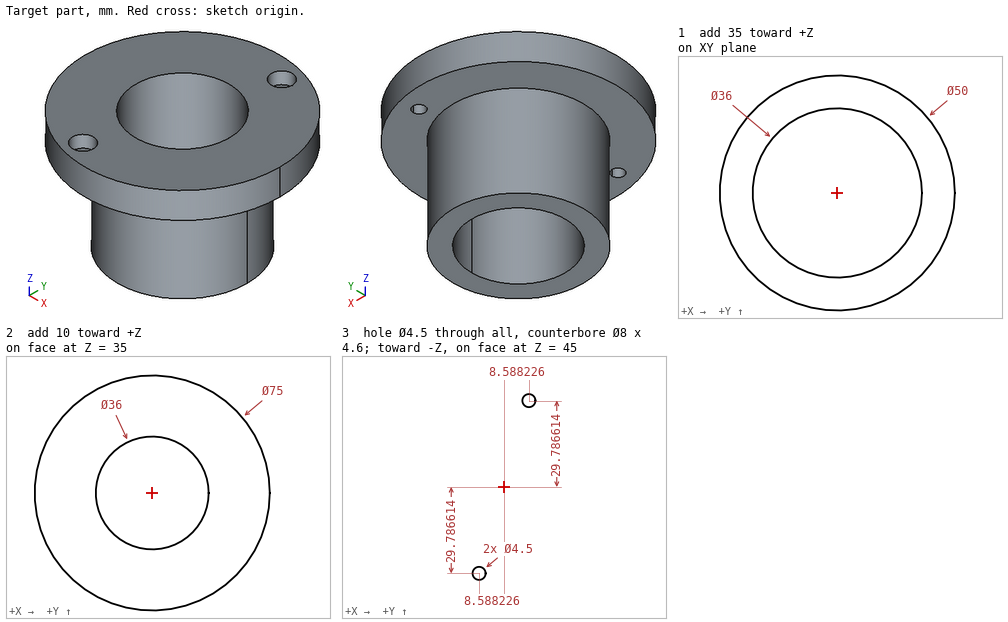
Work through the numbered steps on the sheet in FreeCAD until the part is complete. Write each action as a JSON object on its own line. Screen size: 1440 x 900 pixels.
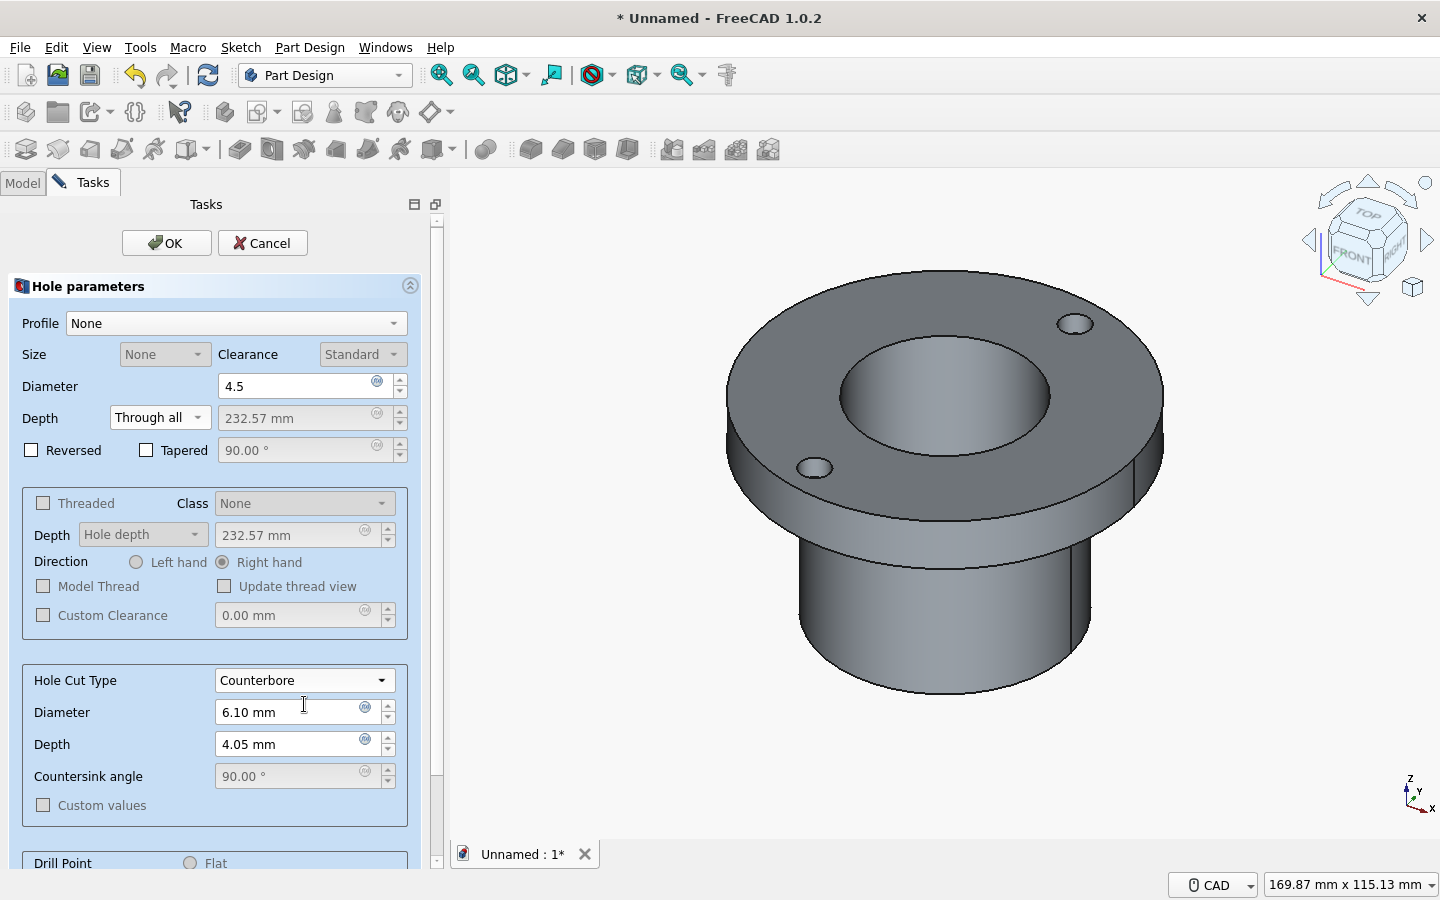
{"action": "triple_click", "coordinate": [298, 712]}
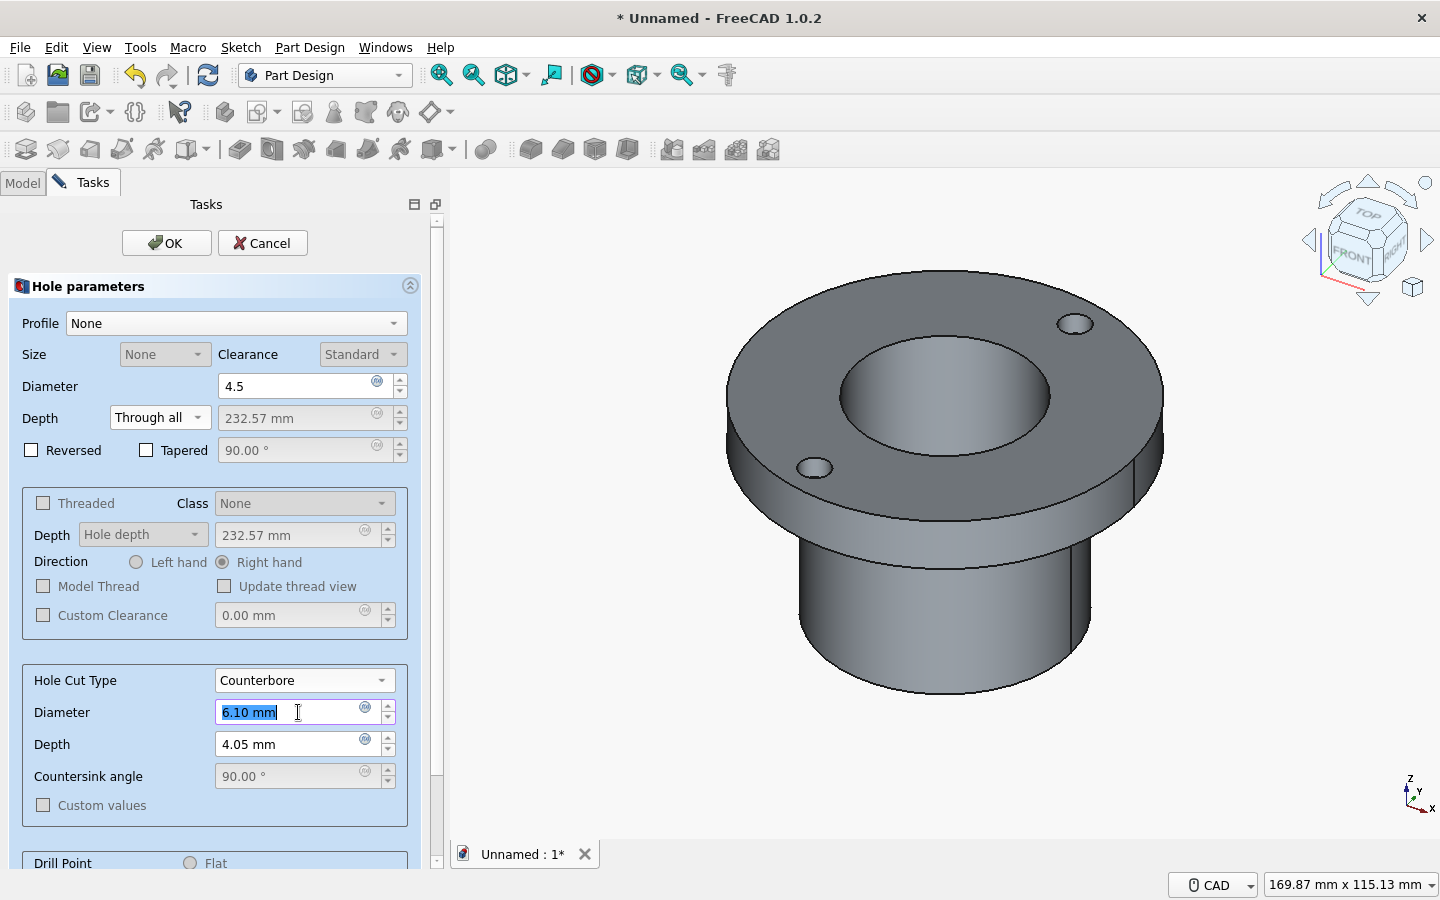
{"action": "type", "text": "8"}
{"action": "key", "text": "Tab"}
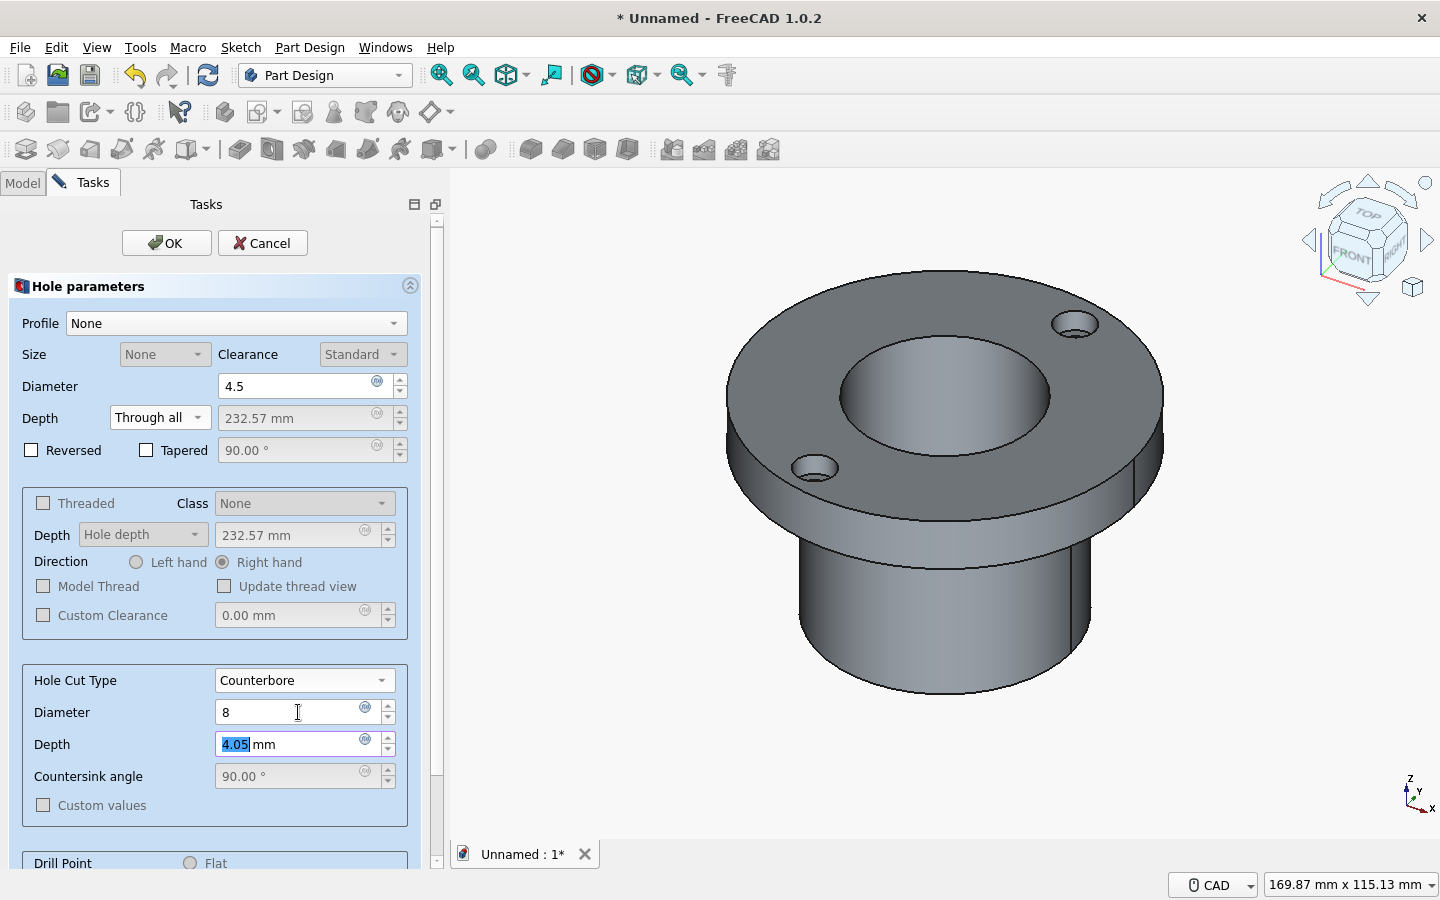
{"action": "type", "text": "4.6"}
{"action": "key", "text": "Tab"}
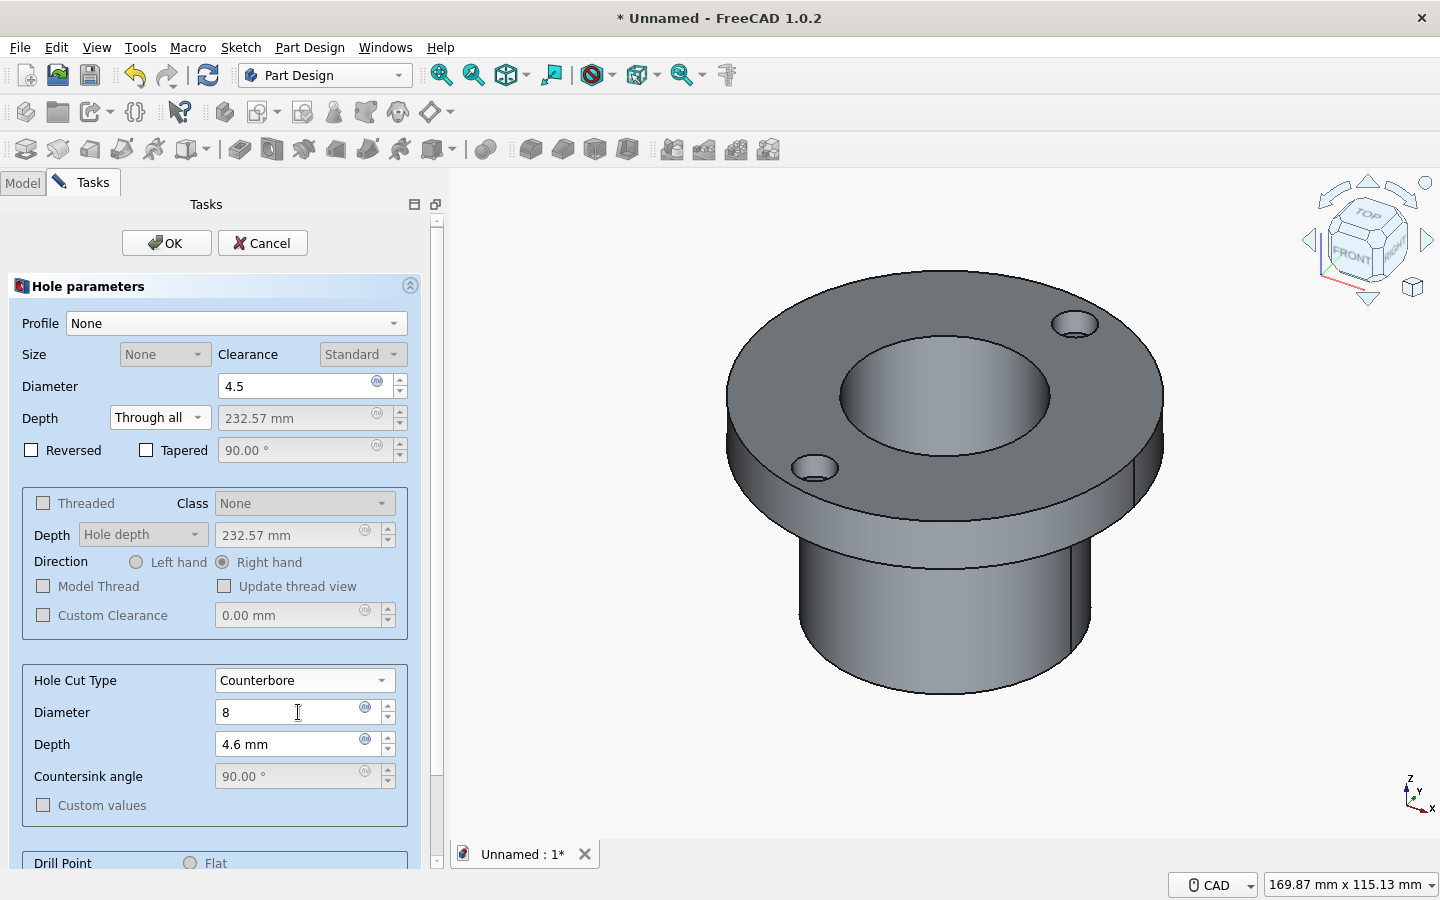
{"action": "left_click", "coordinate": [167, 243]}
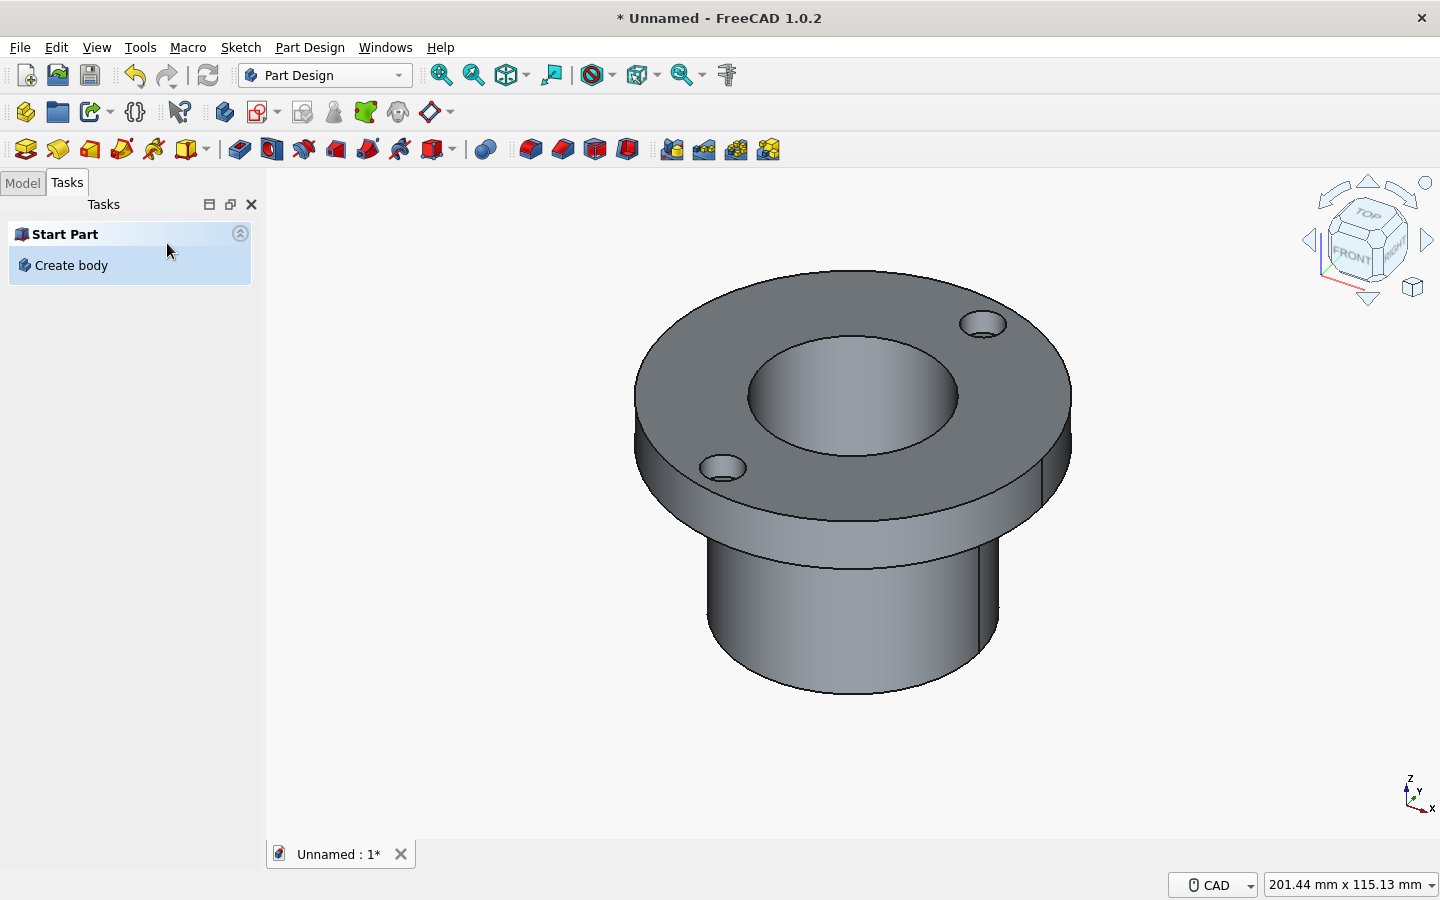
{"action": "key", "text": "0"}